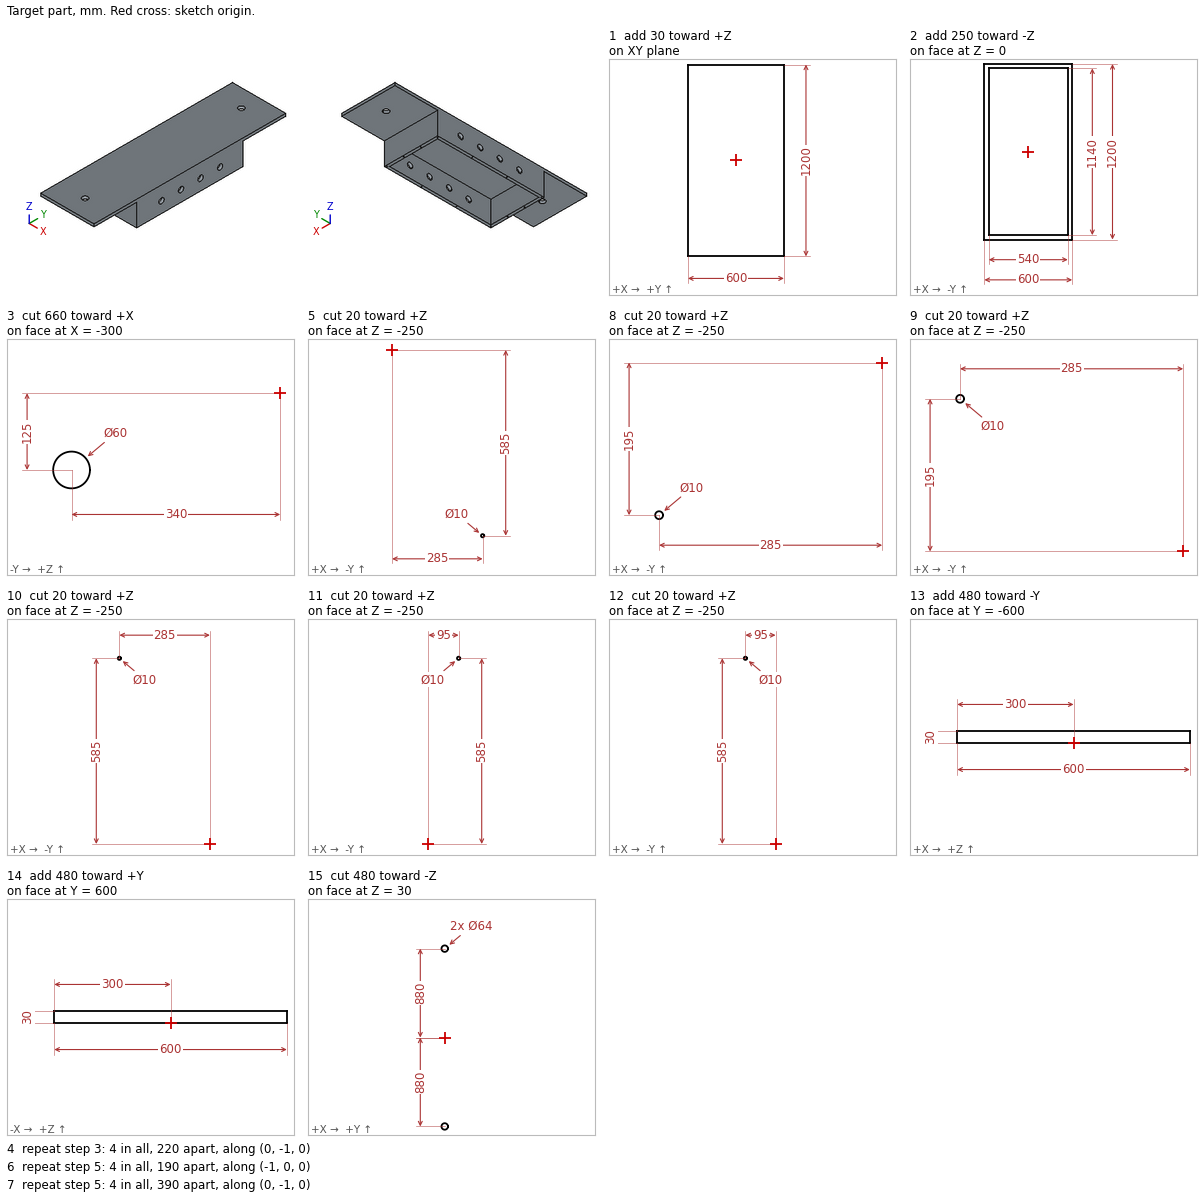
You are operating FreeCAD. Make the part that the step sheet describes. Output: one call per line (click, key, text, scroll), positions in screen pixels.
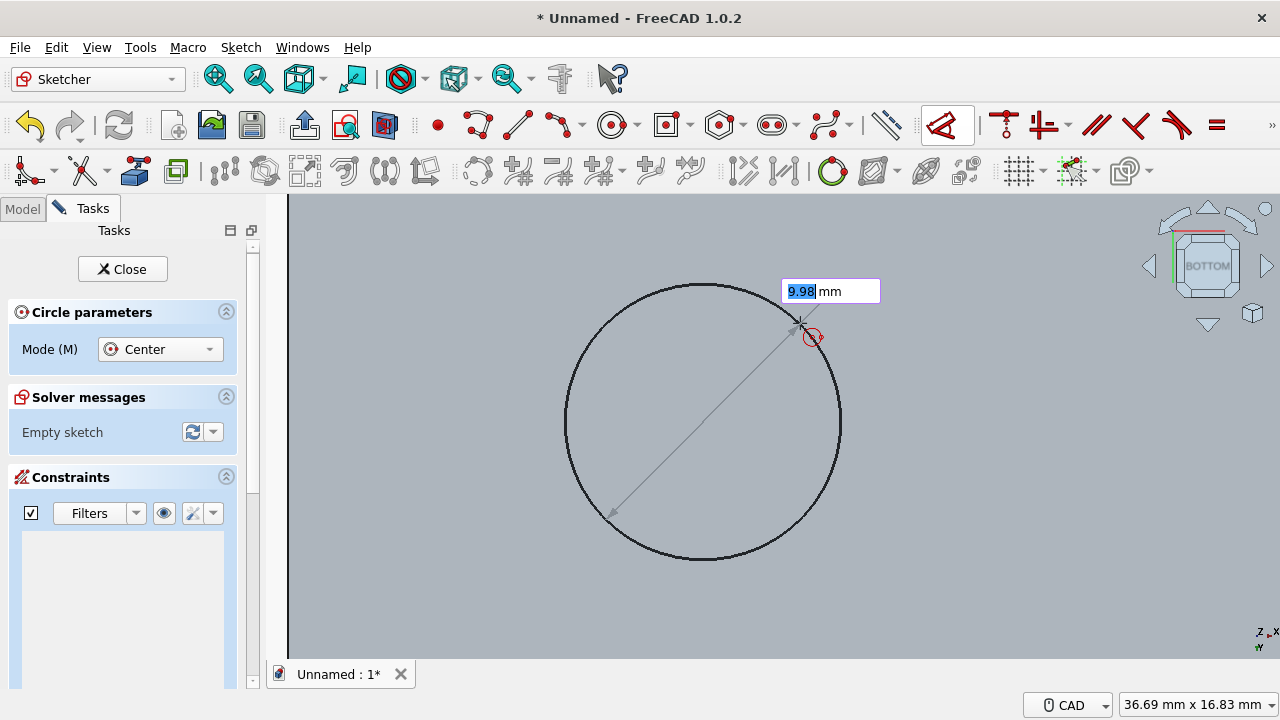
text(10)
key(Return)
key(Escape)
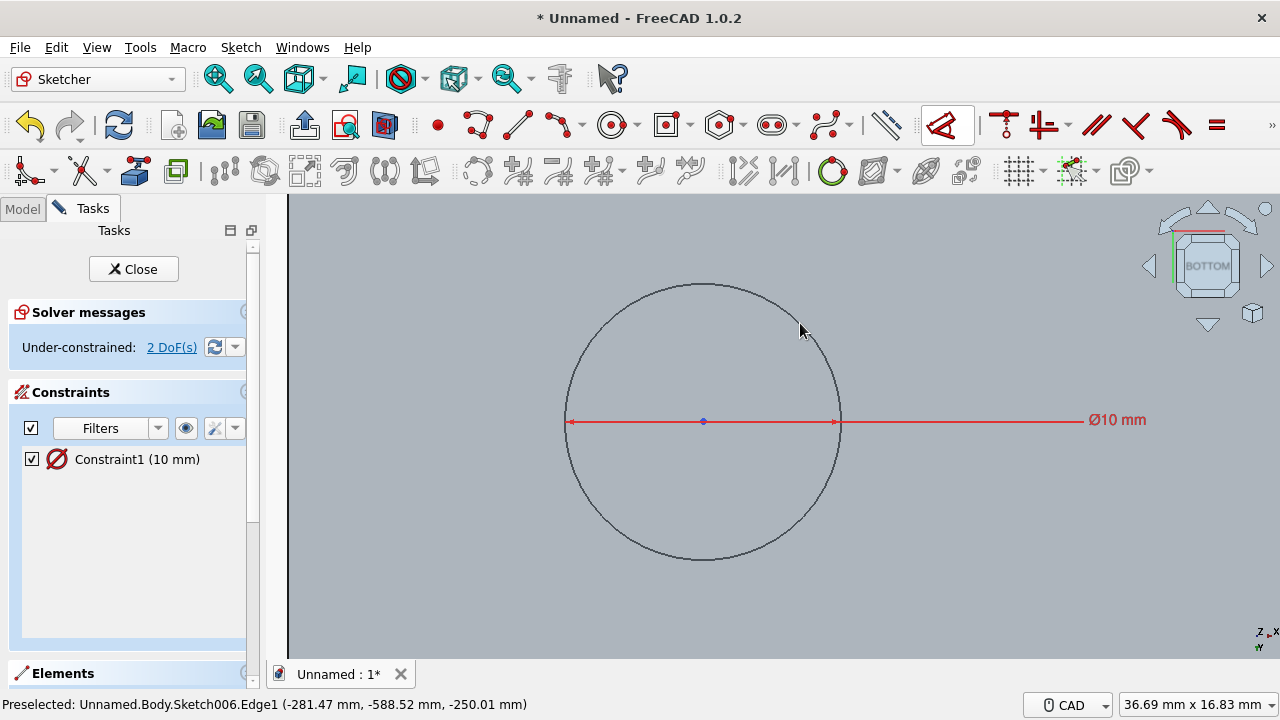
click(703, 422)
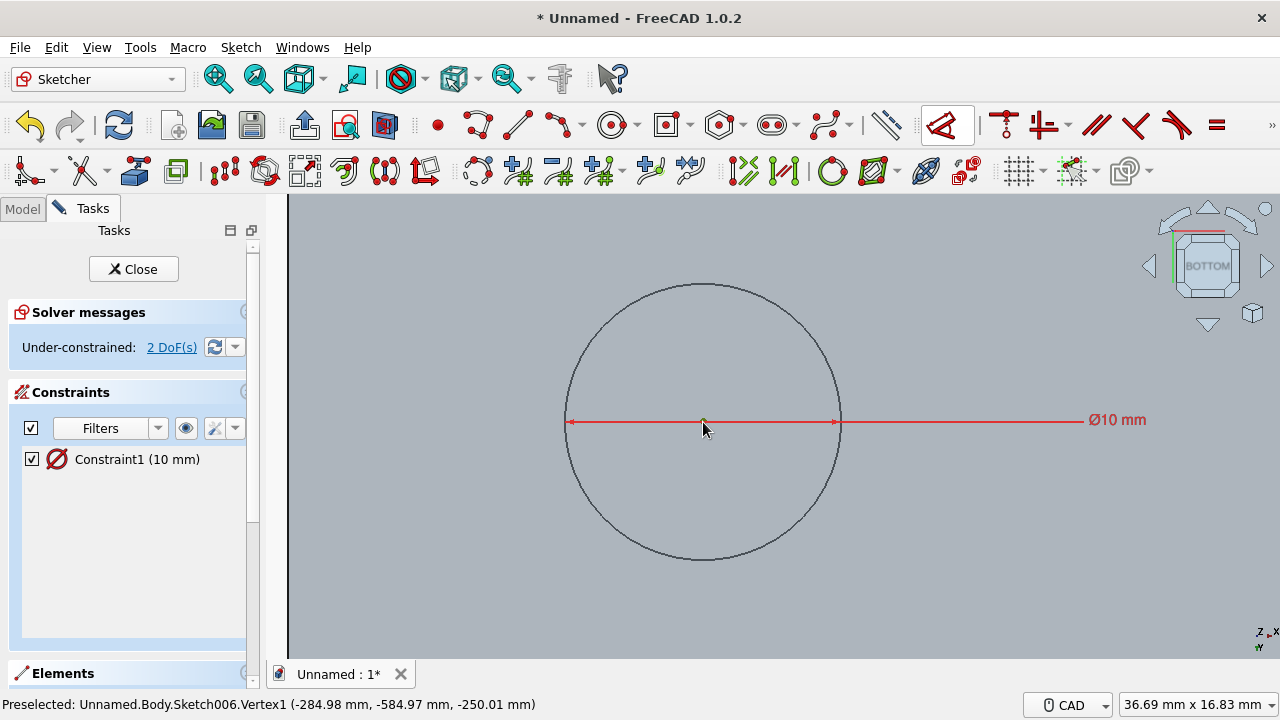
click(968, 126)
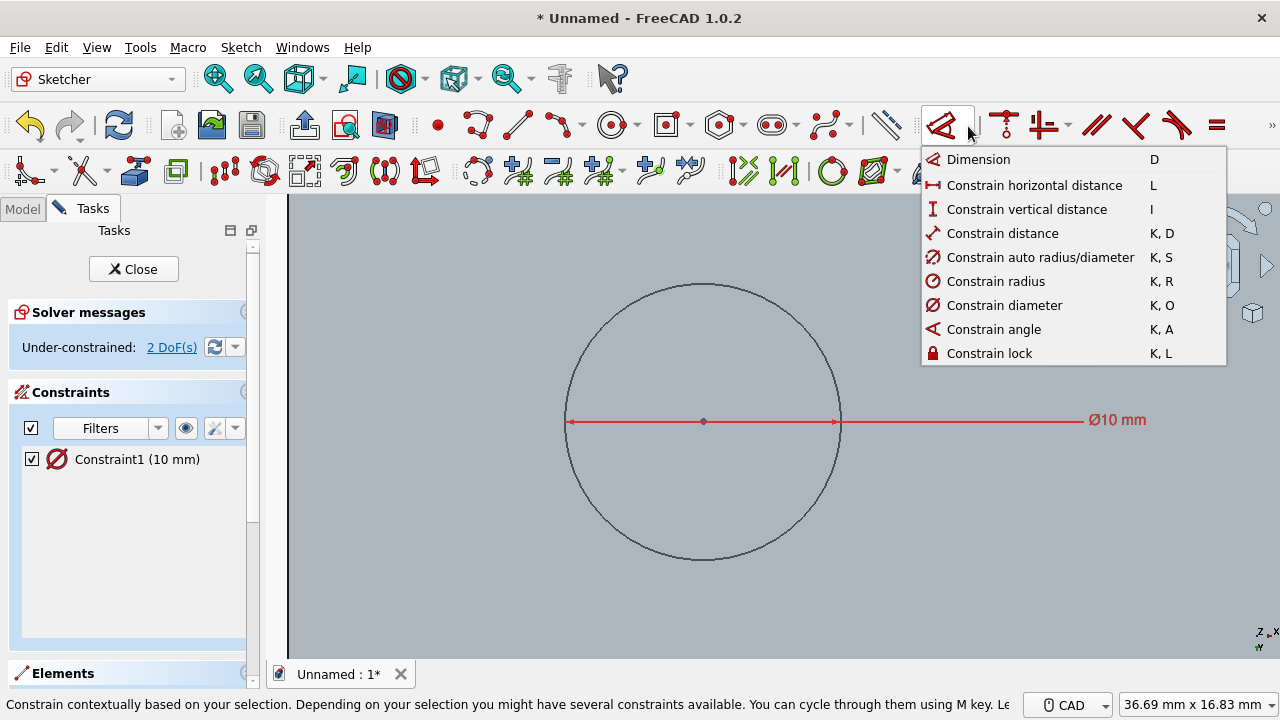
click(1074, 185)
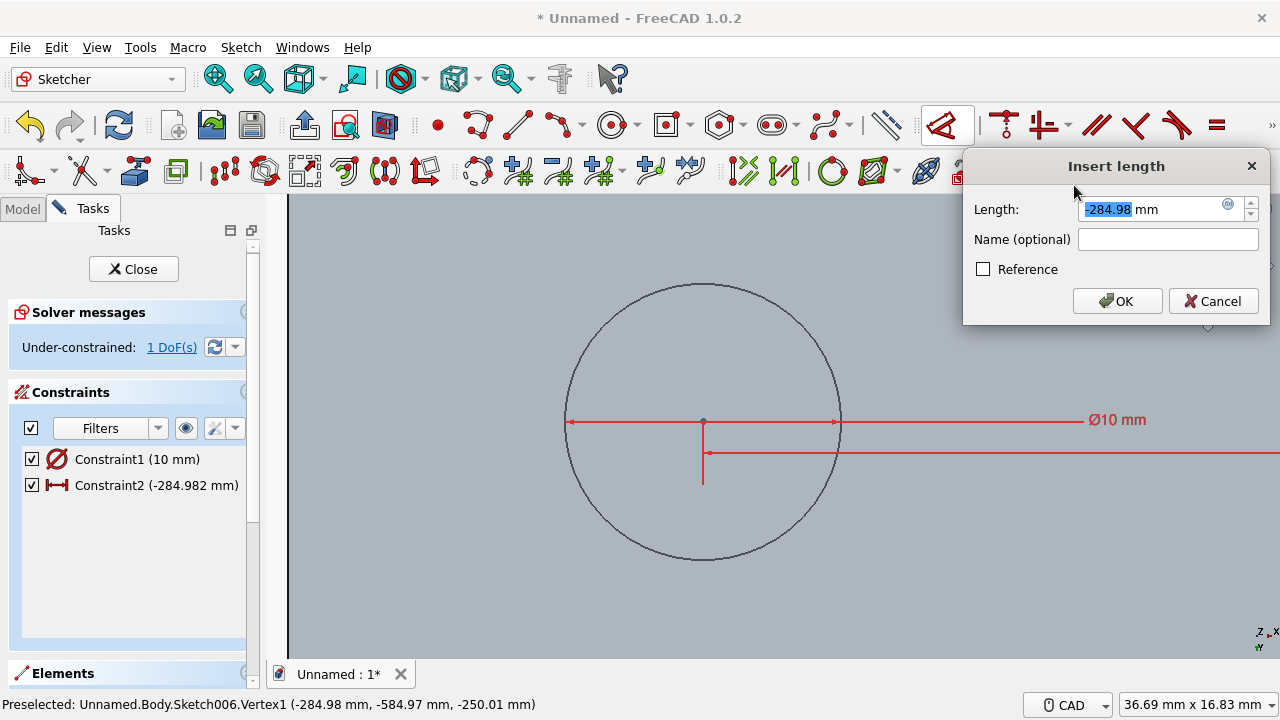
text(-285)
key(Return)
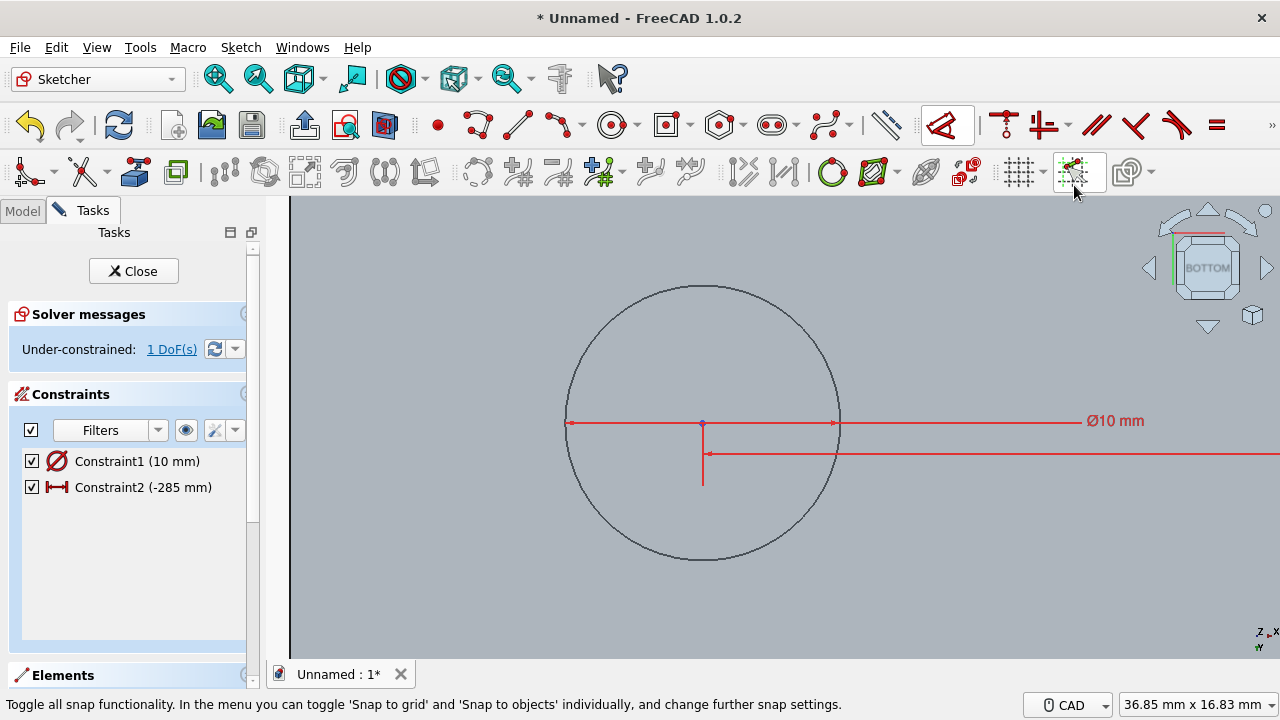
click(703, 423)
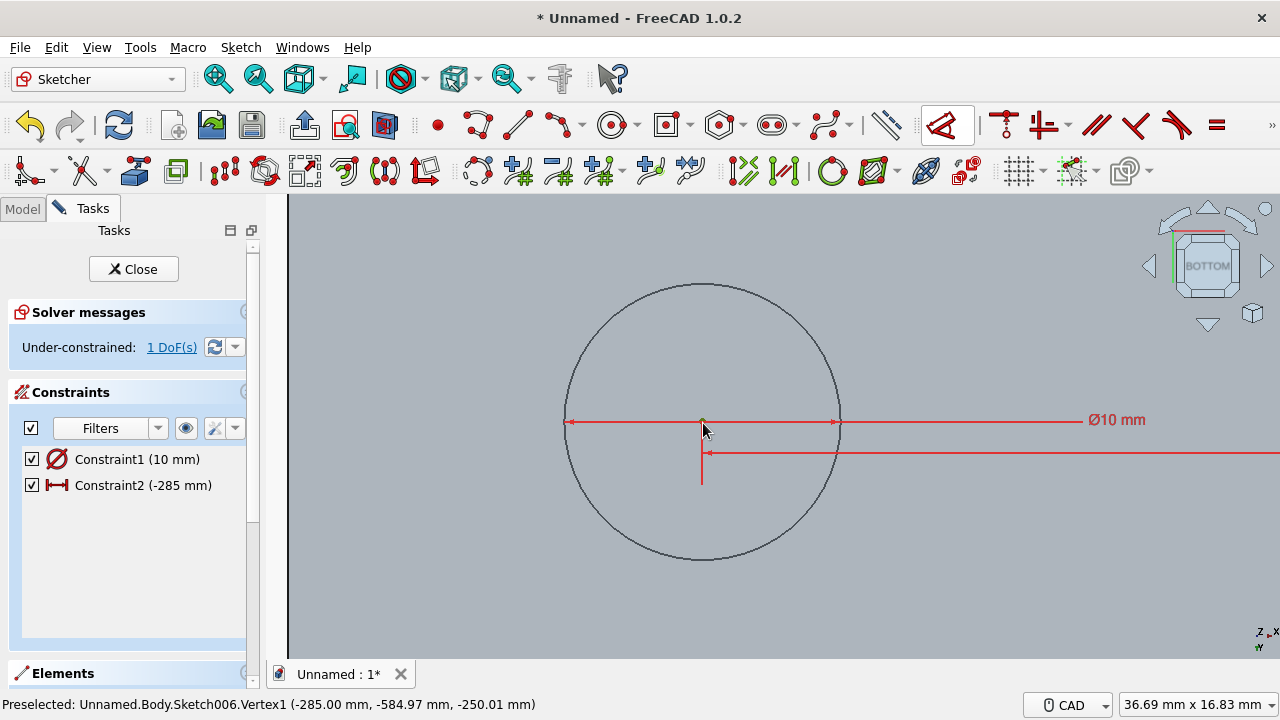
click(968, 126)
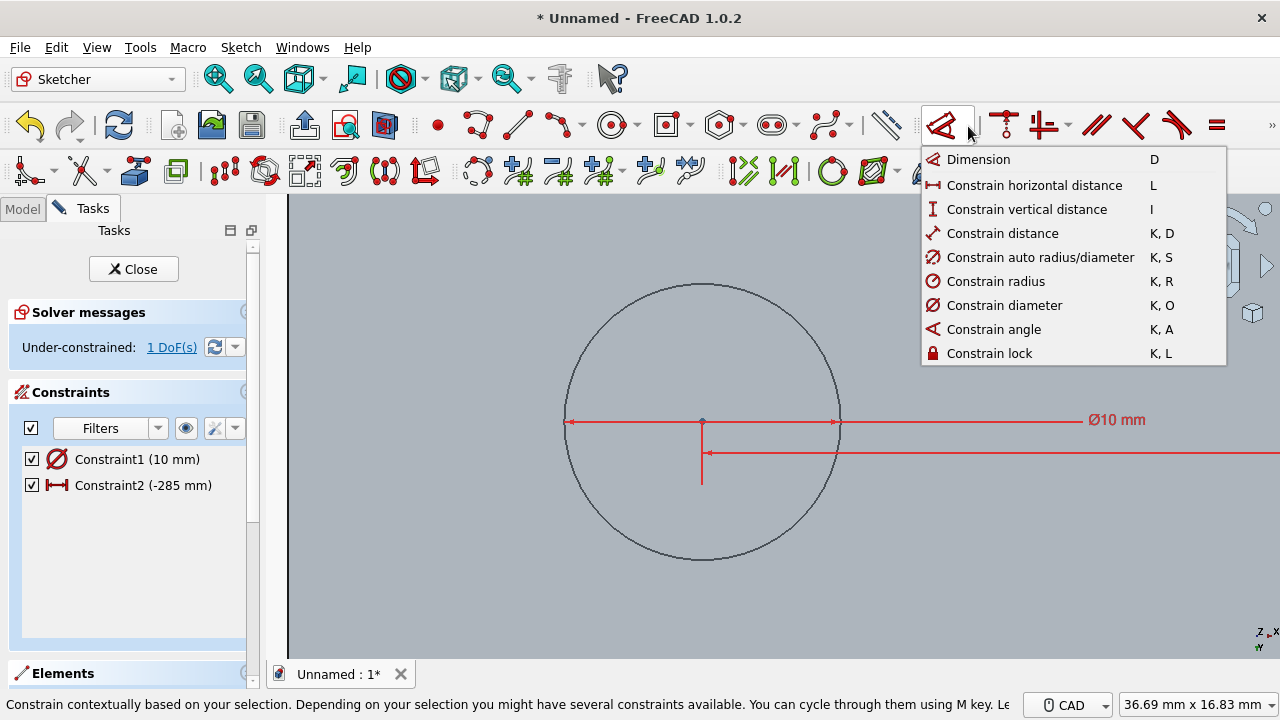
click(1074, 209)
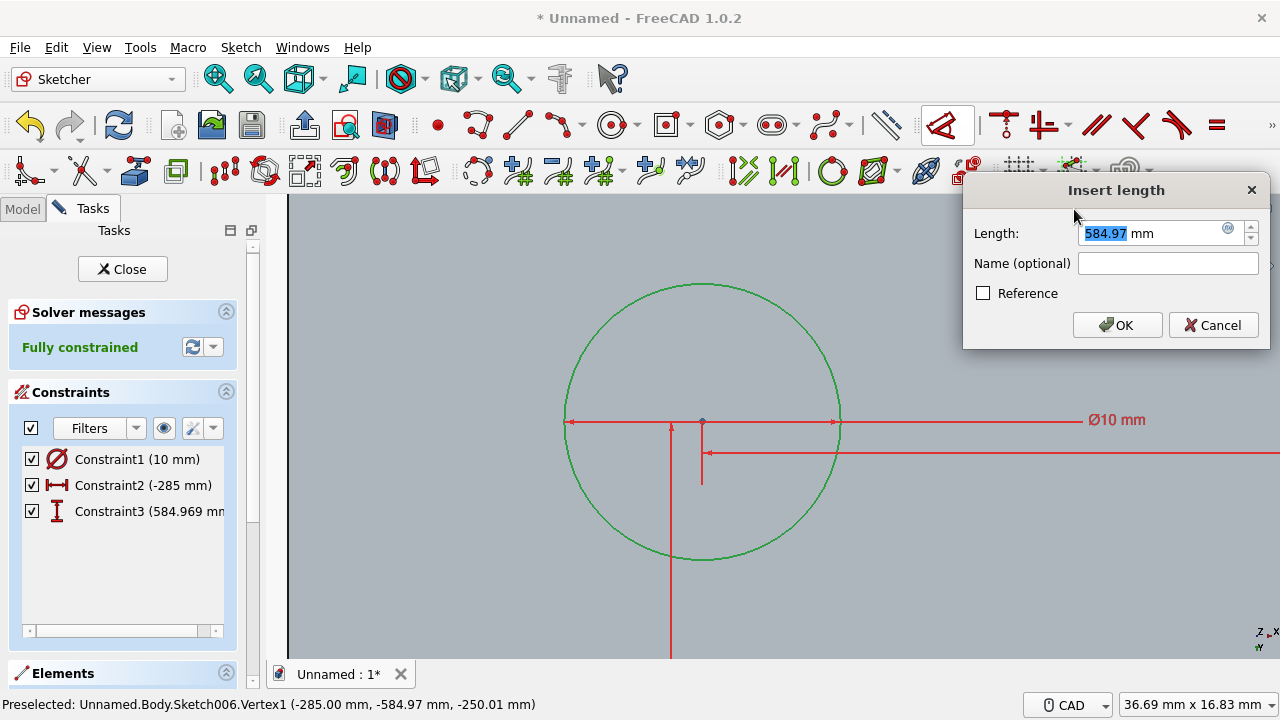
text(585)
key(Return)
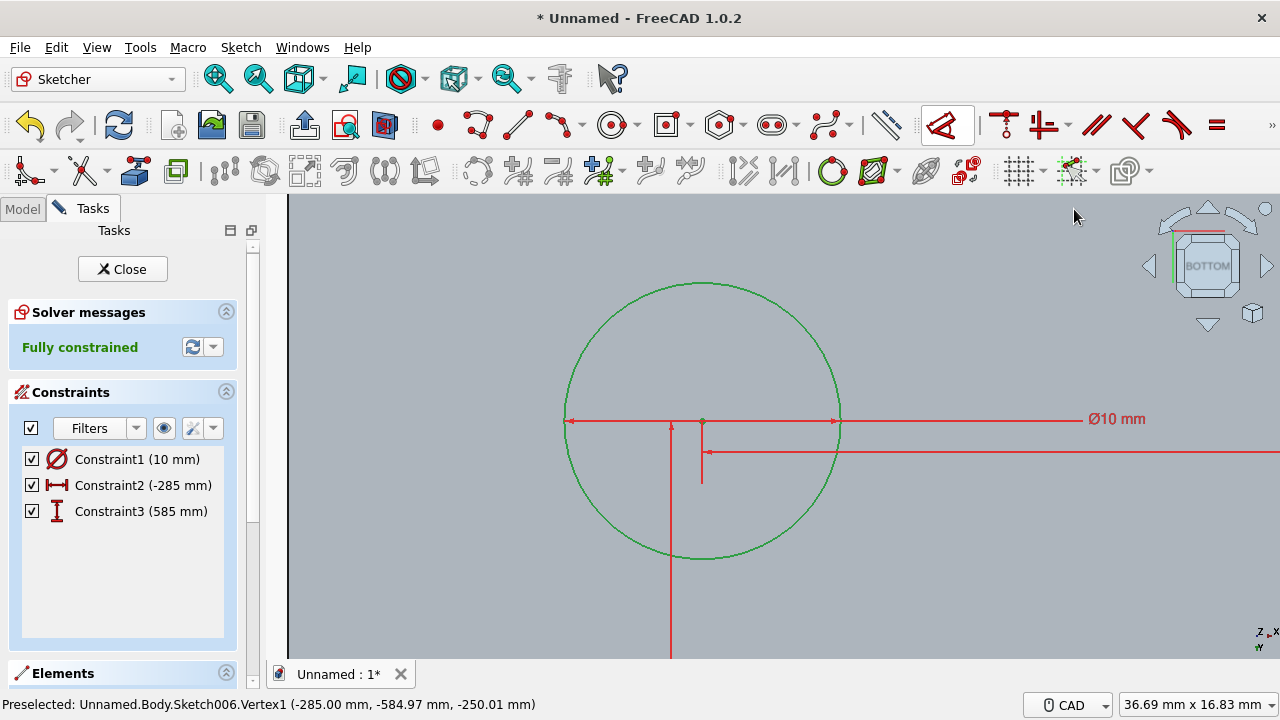
click(123, 269)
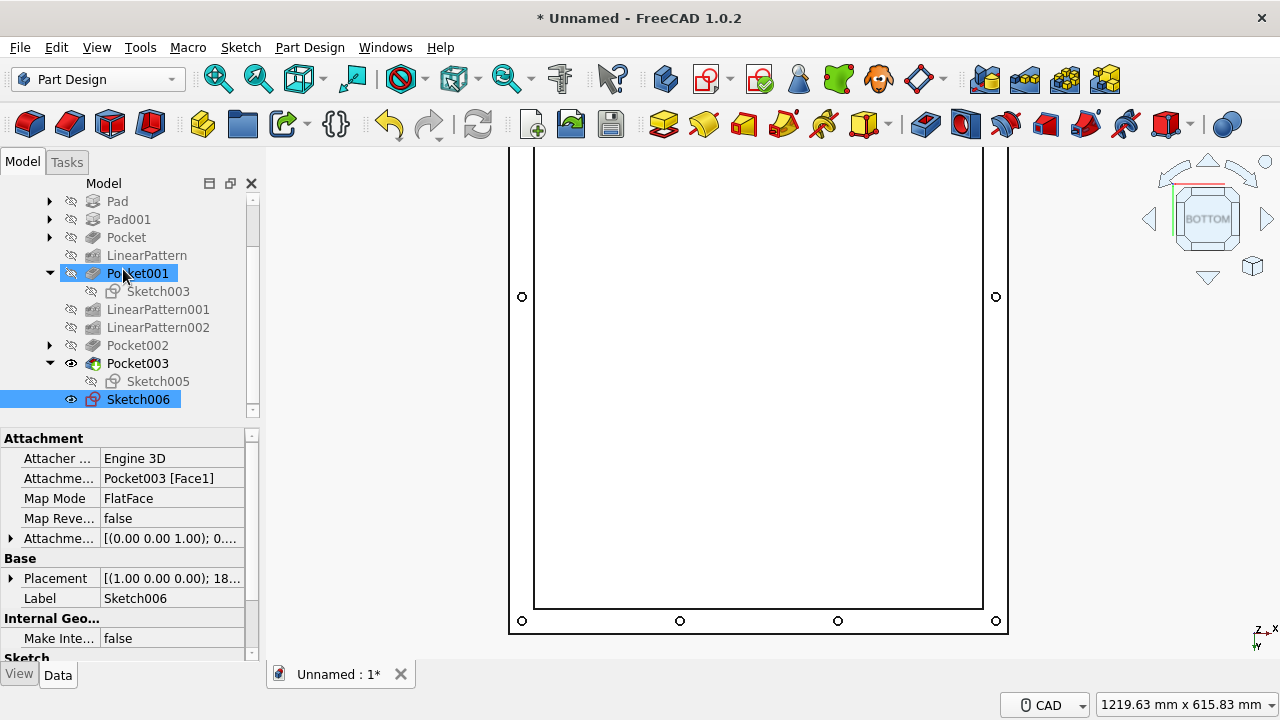
click(926, 124)